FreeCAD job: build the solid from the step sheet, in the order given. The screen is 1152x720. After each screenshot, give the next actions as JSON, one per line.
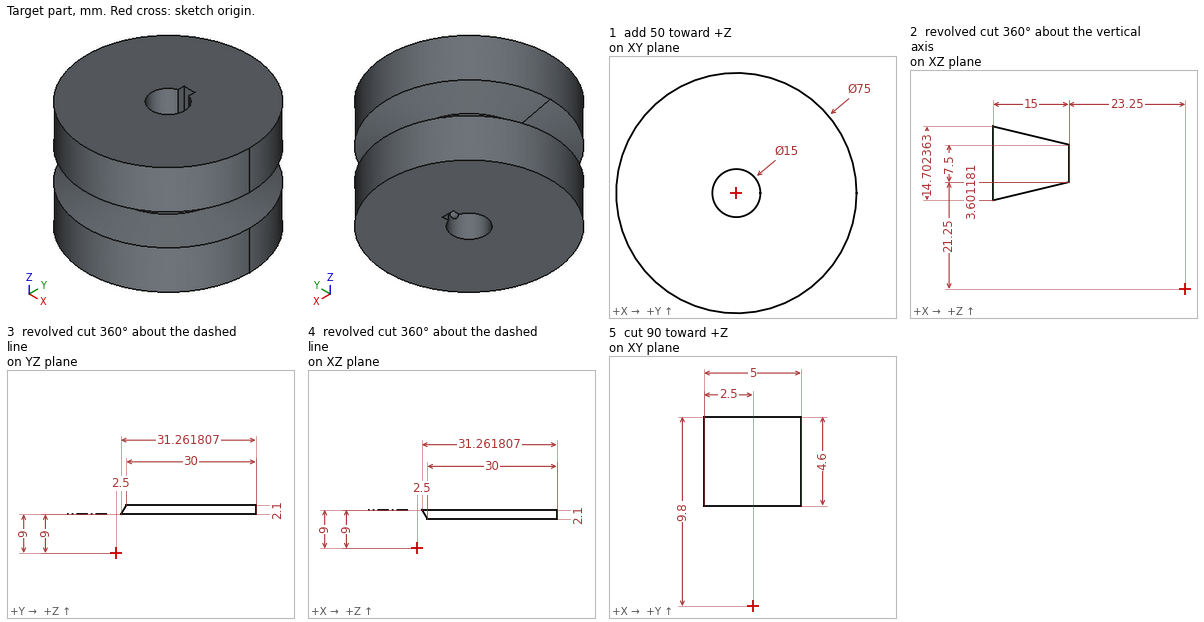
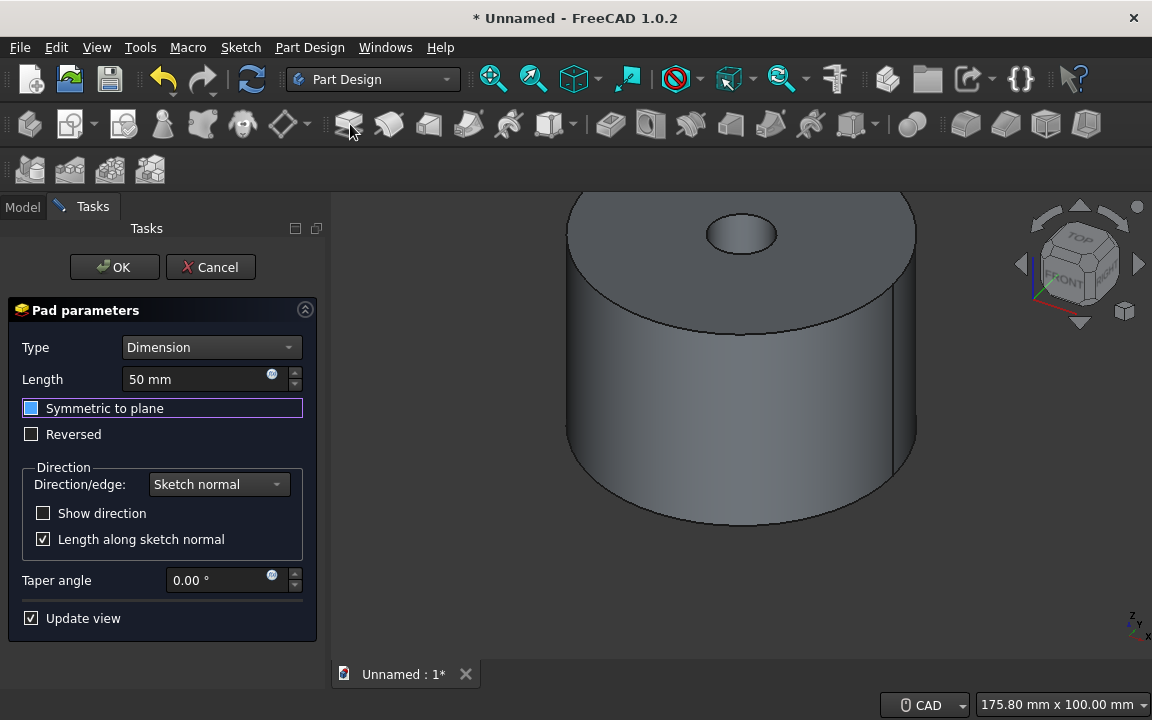
{"action": "left_click", "coordinate": [115, 267]}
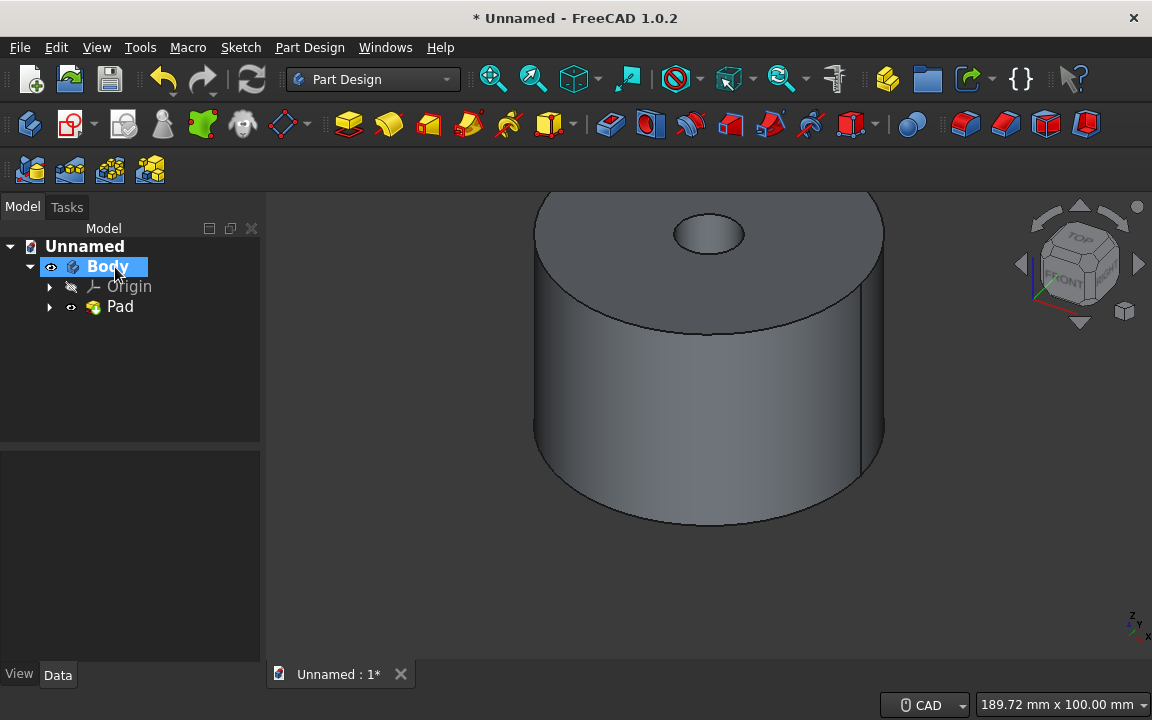
{"action": "left_click", "coordinate": [494, 80]}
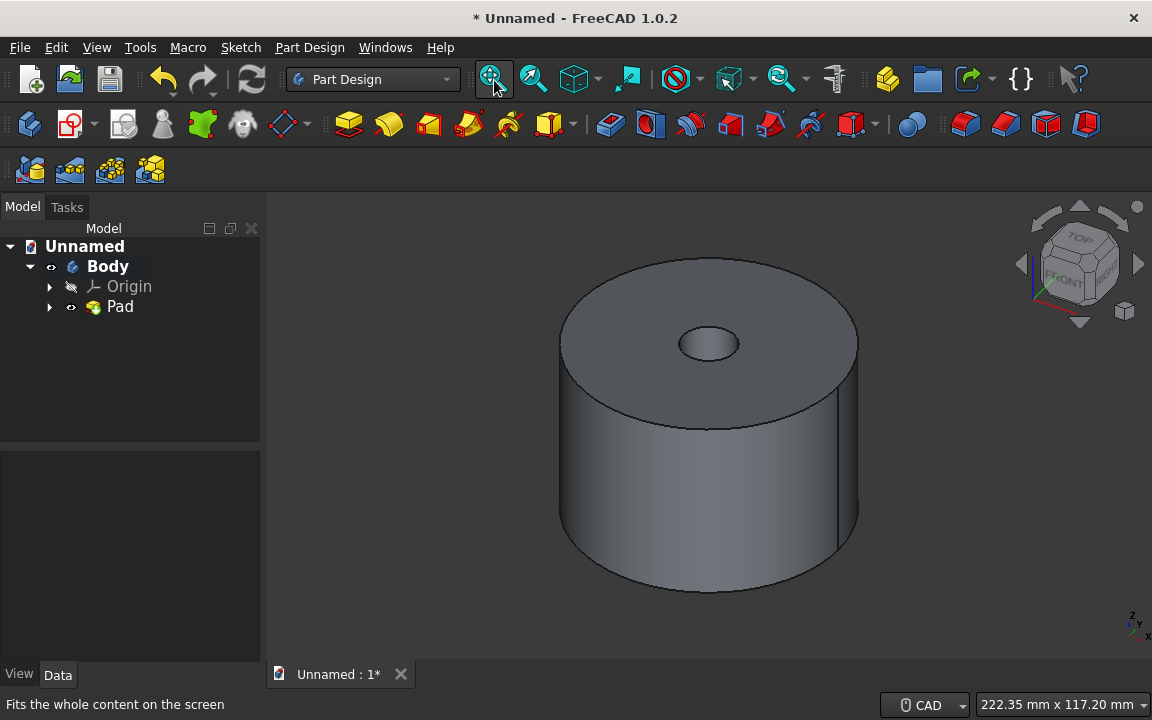
{"action": "left_click", "coordinate": [70, 124]}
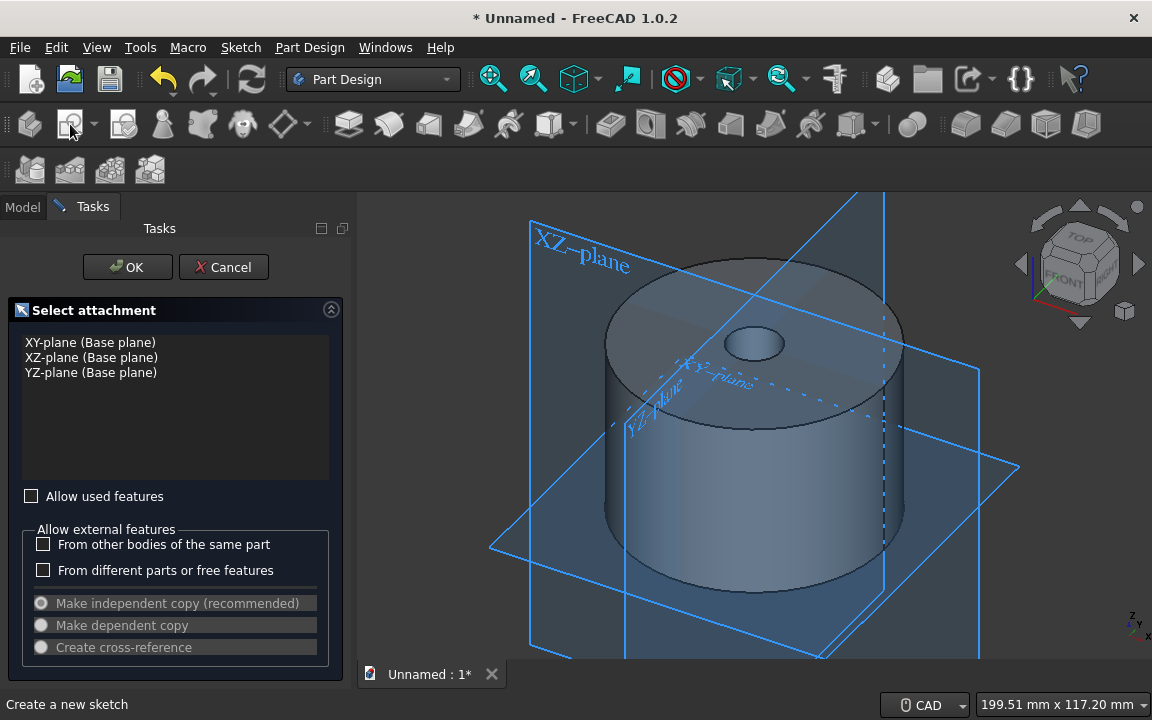
{"action": "left_click", "coordinate": [82, 358]}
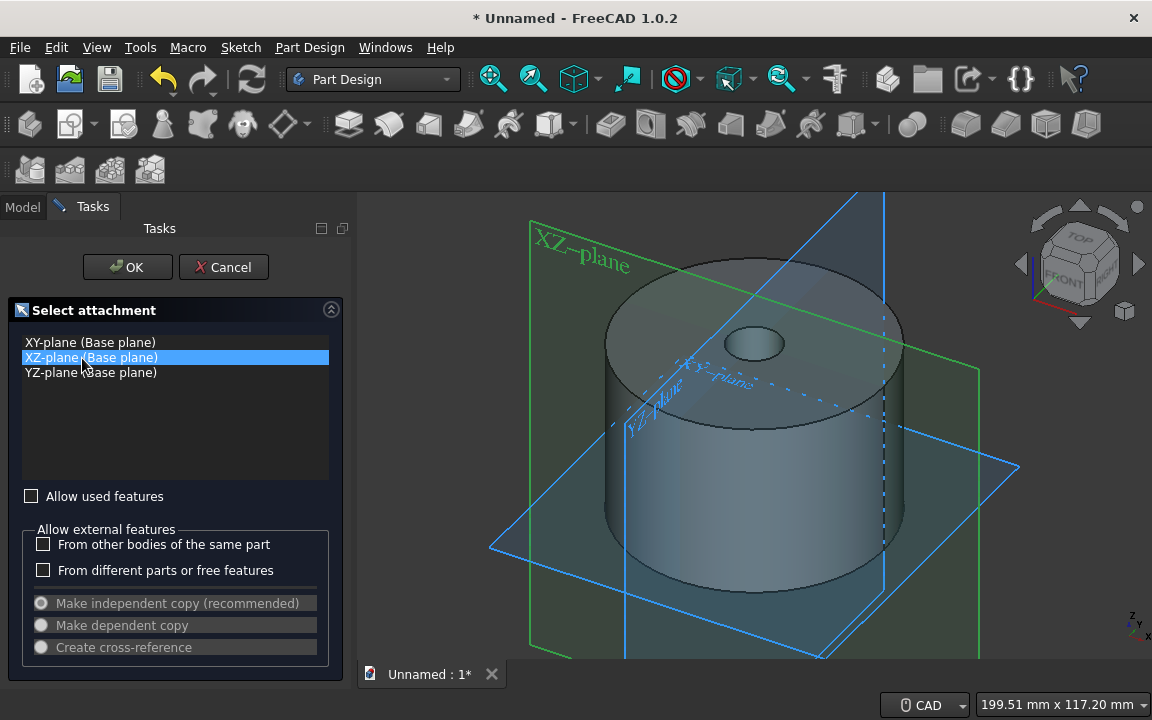
{"action": "left_click", "coordinate": [128, 267]}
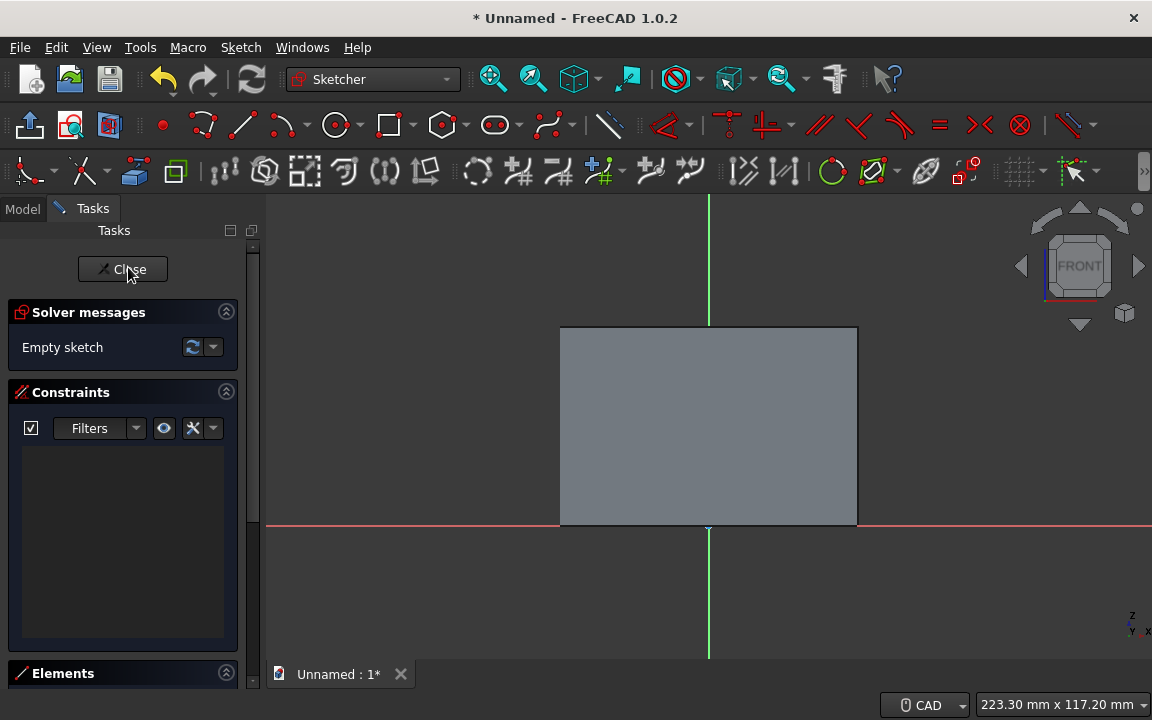
{"action": "left_click", "coordinate": [110, 126]}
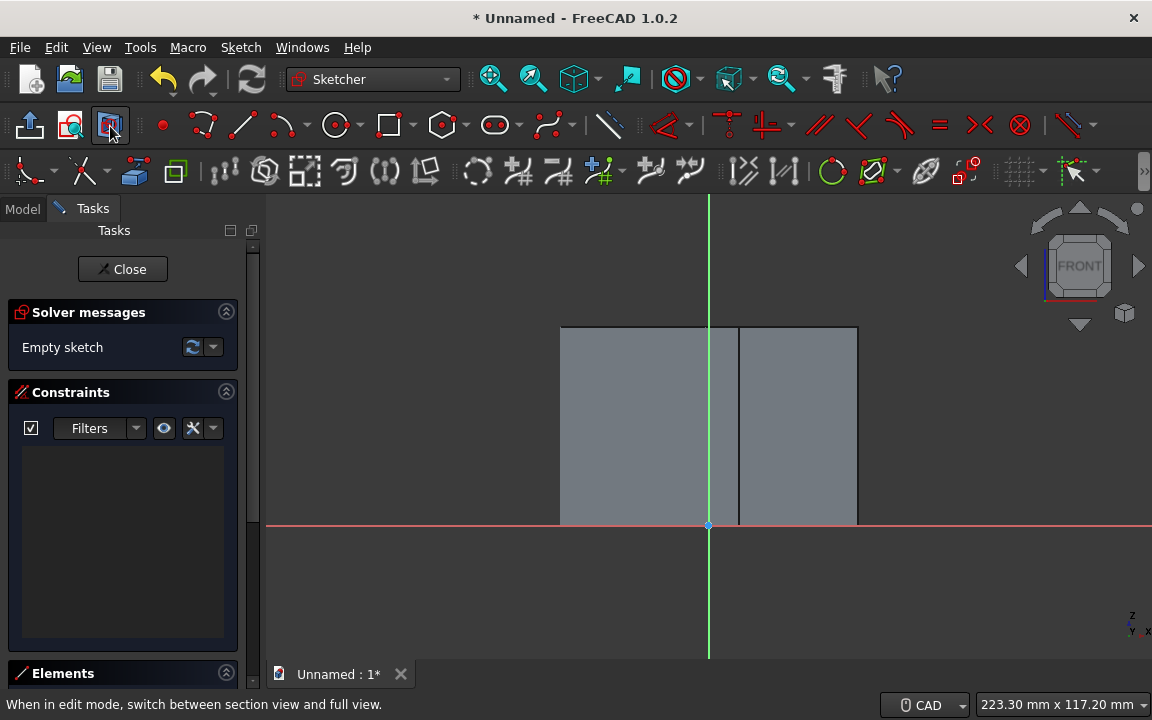
{"action": "scroll", "coordinate": [573, 427], "scroll_direction": "up", "scroll_amount": 8}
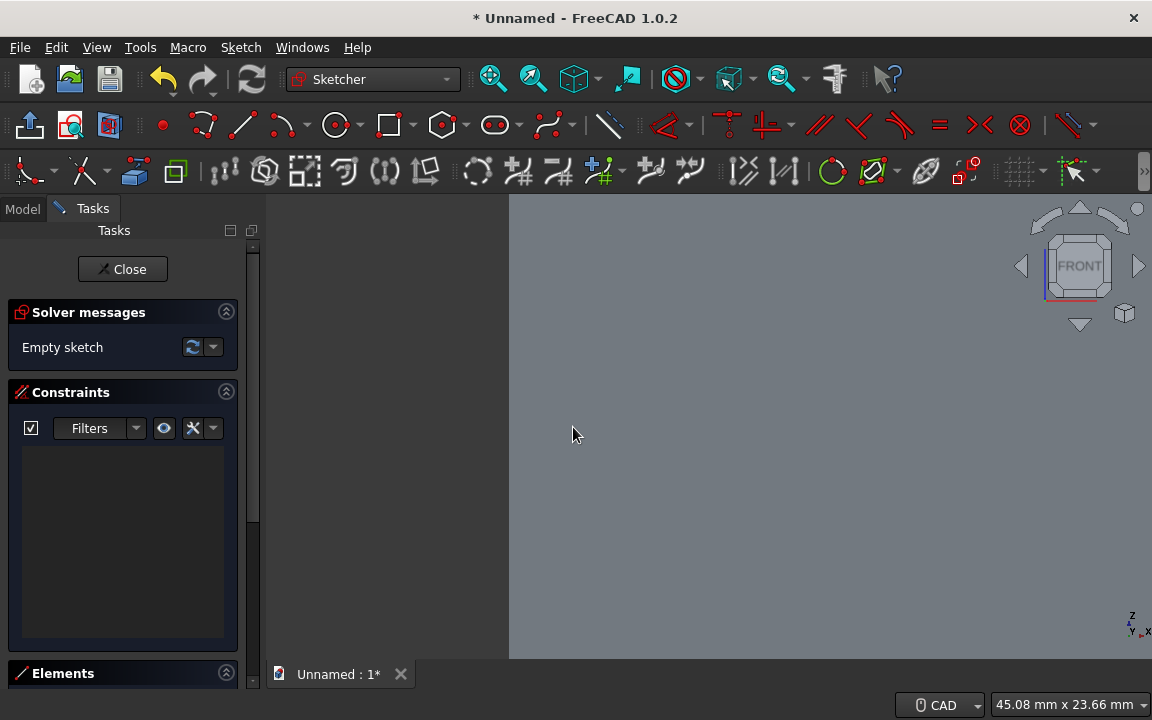
{"action": "left_click", "coordinate": [204, 126]}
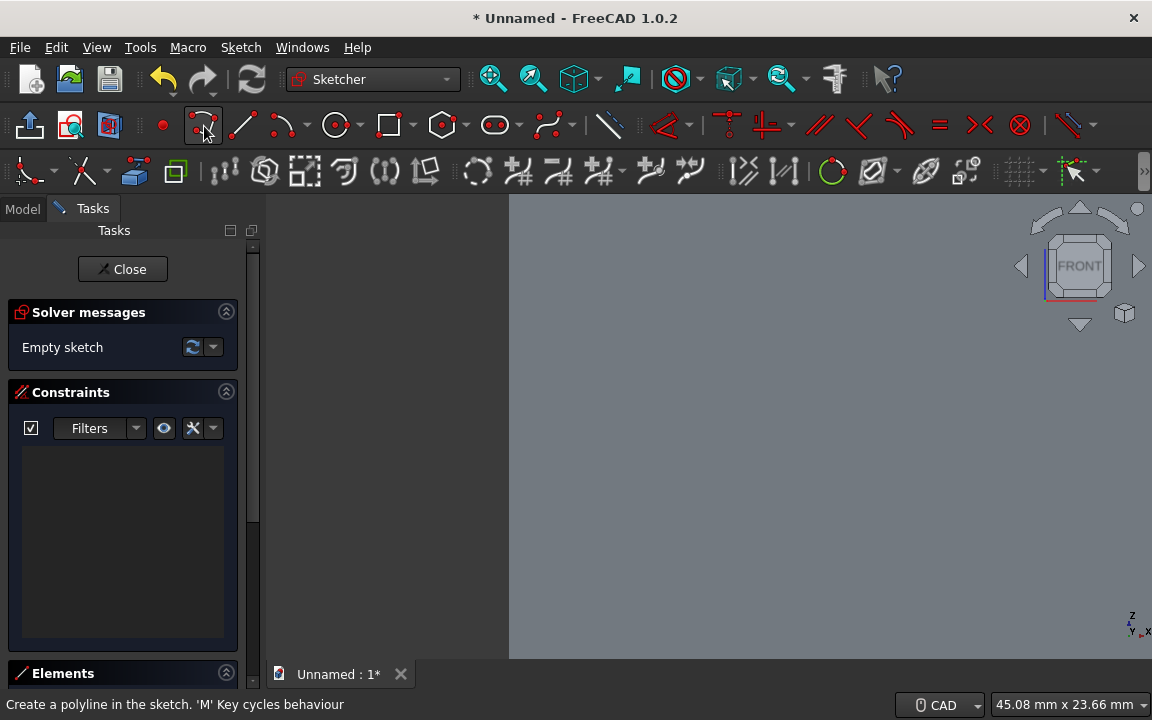
{"action": "left_click", "coordinate": [788, 496]}
{"action": "left_click", "coordinate": [493, 567]}
{"action": "left_click", "coordinate": [493, 278]}
{"action": "left_click", "coordinate": [788, 349]}
{"action": "left_click", "coordinate": [788, 497]}
{"action": "key", "text": "Escape"}
{"action": "key", "text": "Escape"}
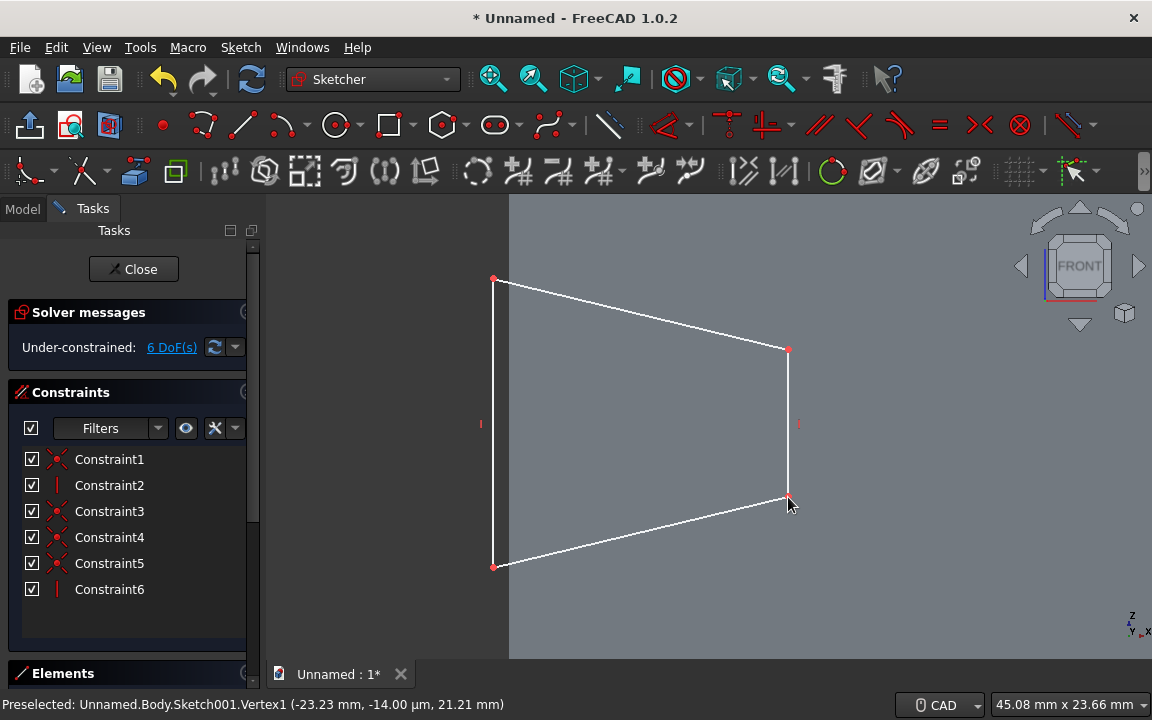
{"action": "left_click", "coordinate": [664, 126]}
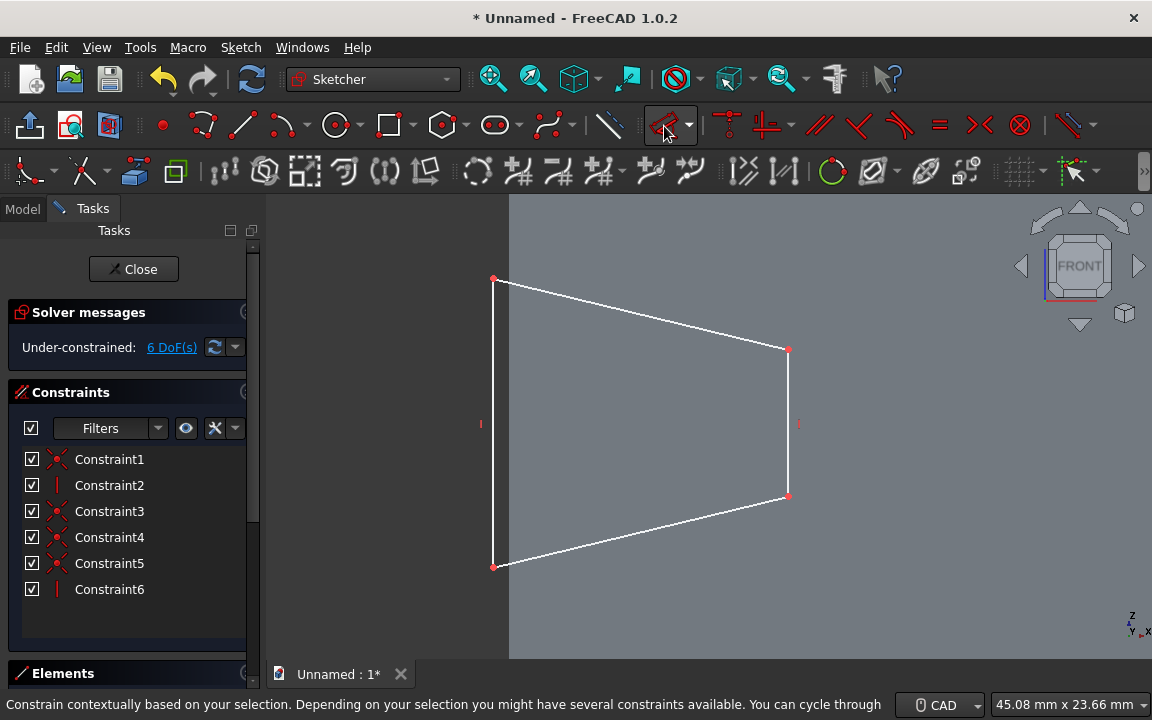
{"action": "left_click", "coordinate": [788, 394]}
{"action": "left_click", "coordinate": [822, 423]}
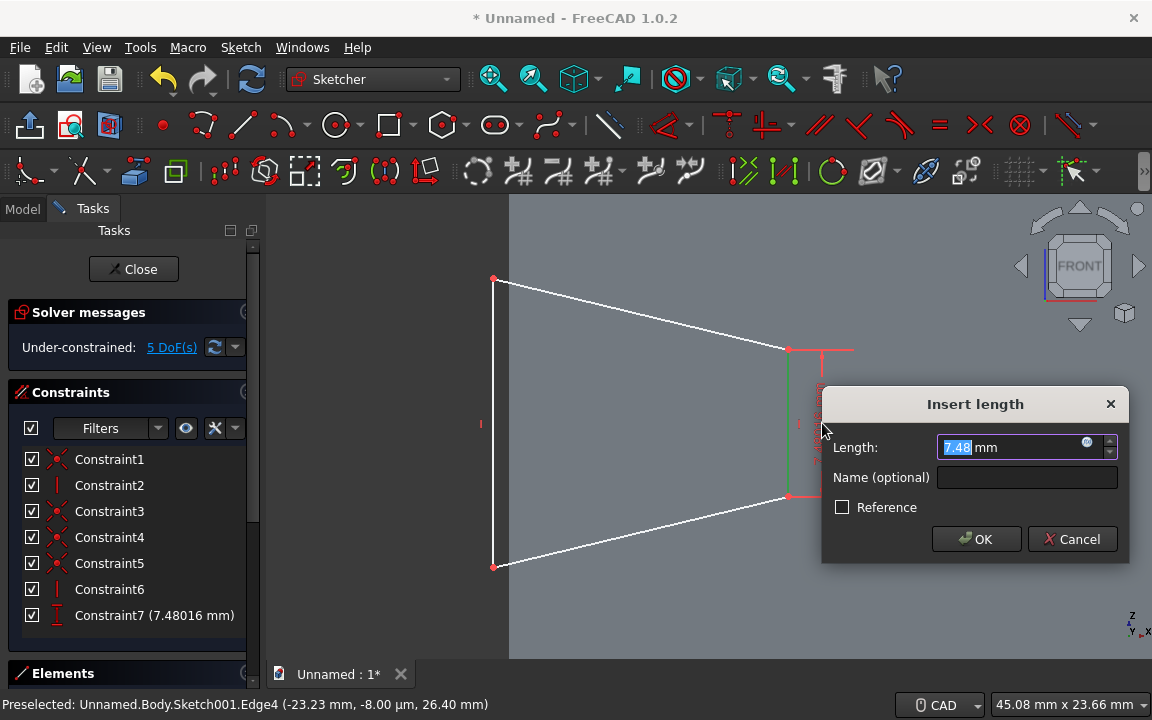
{"action": "type", "text": "7.5"}
{"action": "key", "text": "Return"}